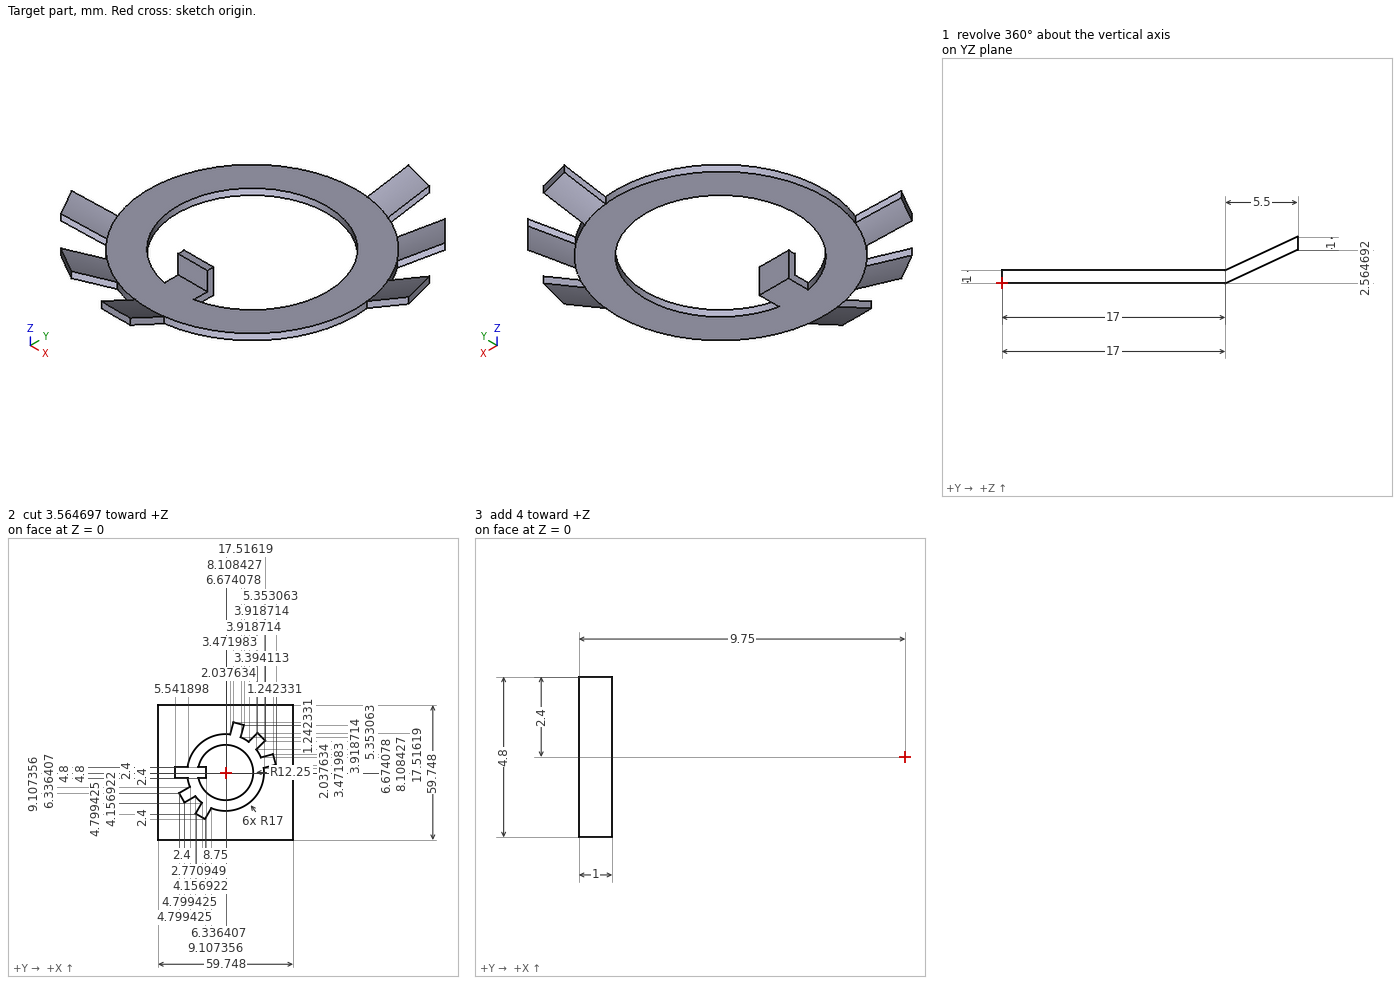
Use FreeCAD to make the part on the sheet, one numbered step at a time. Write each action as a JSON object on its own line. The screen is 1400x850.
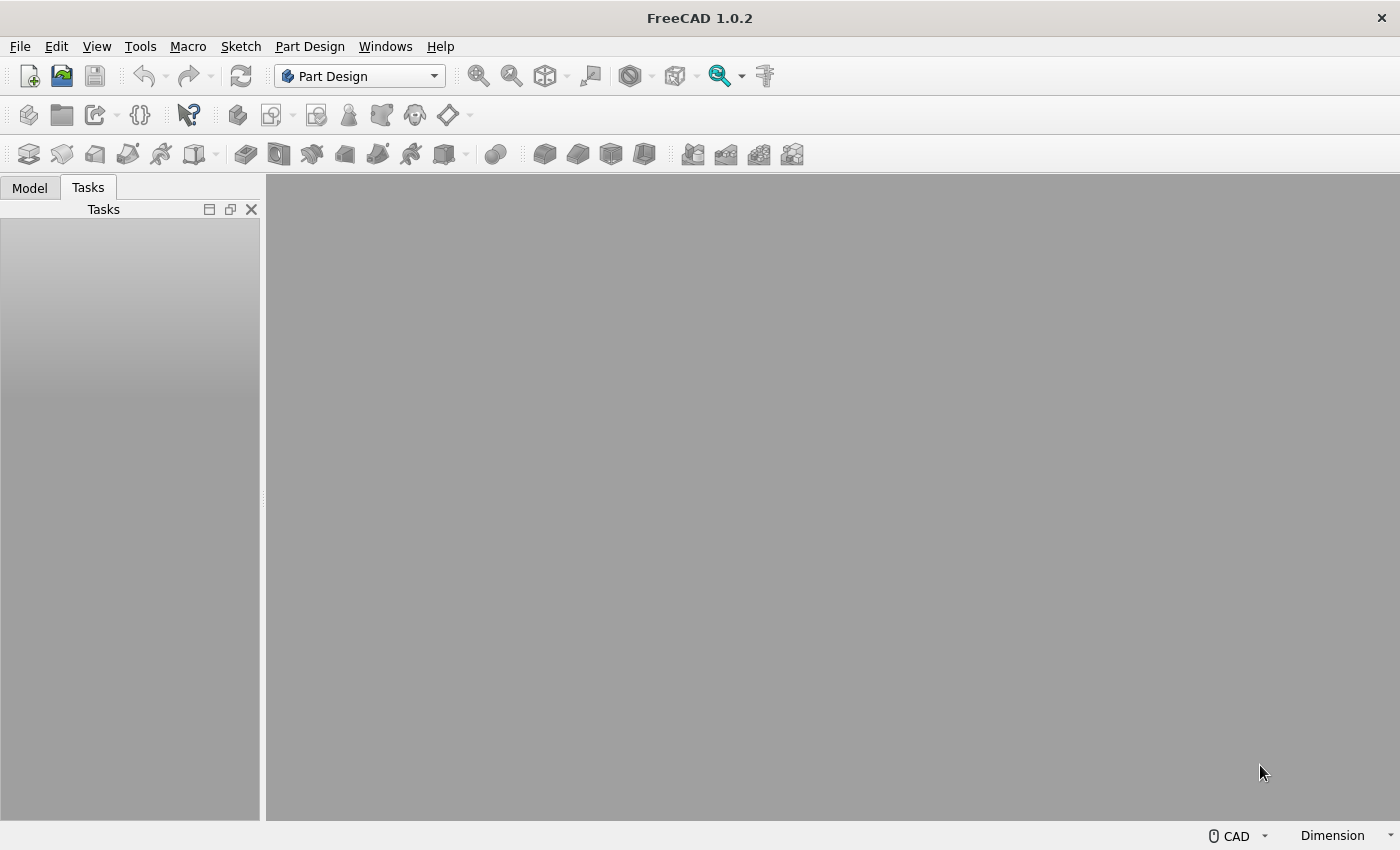
{"action": "left_click", "coordinate": [29, 76]}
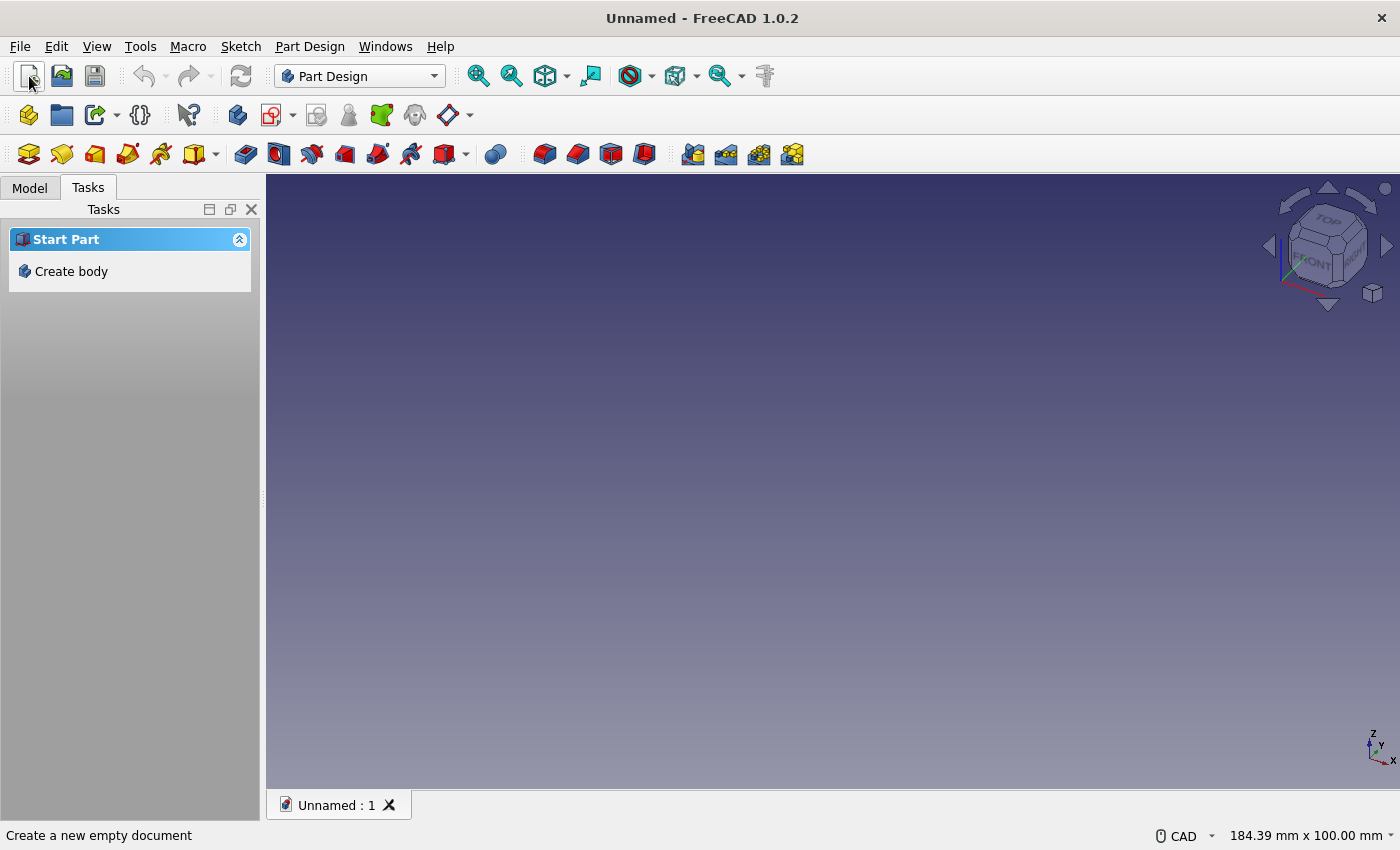
{"action": "left_click", "coordinate": [270, 116]}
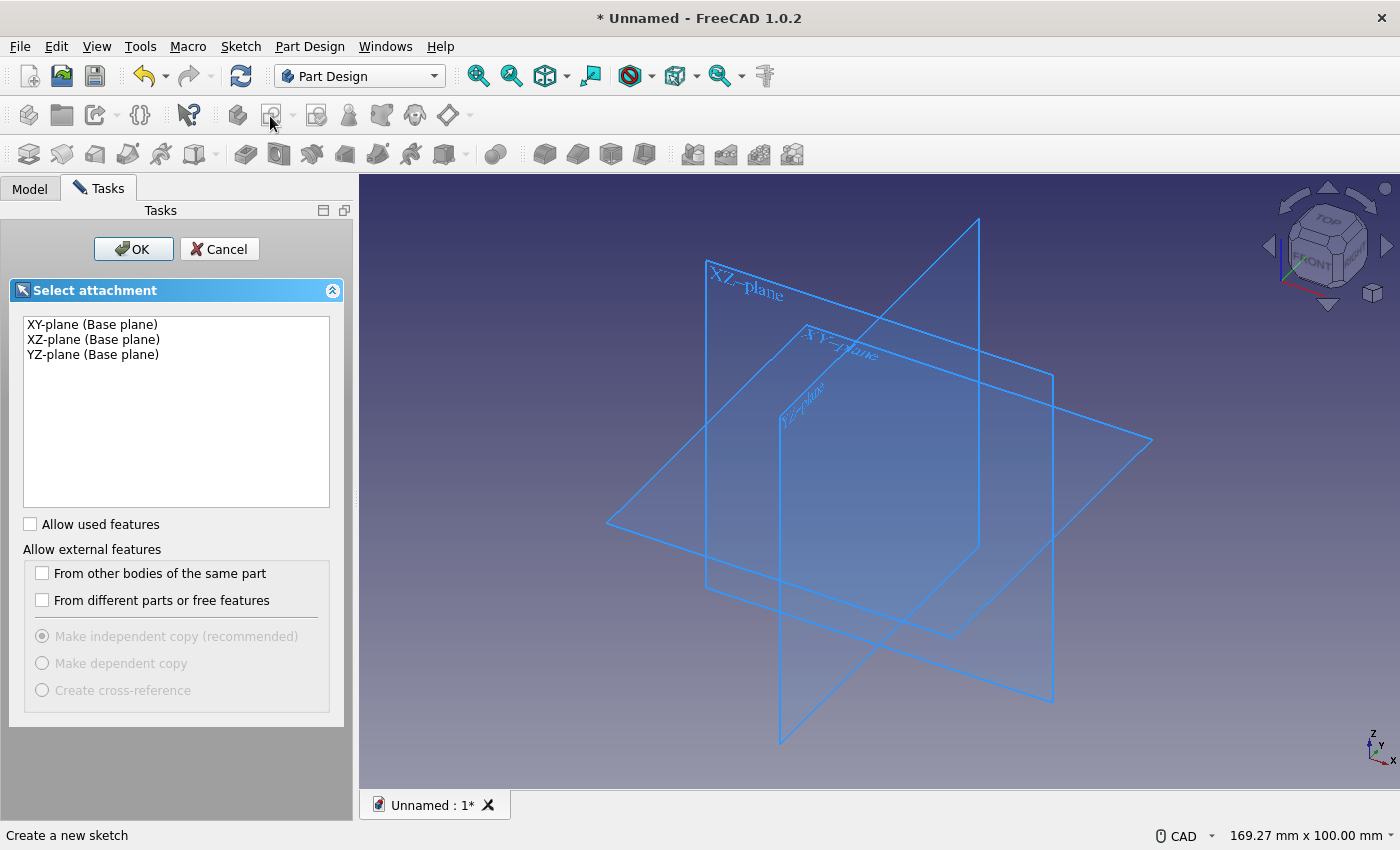
{"action": "left_click", "coordinate": [84, 354]}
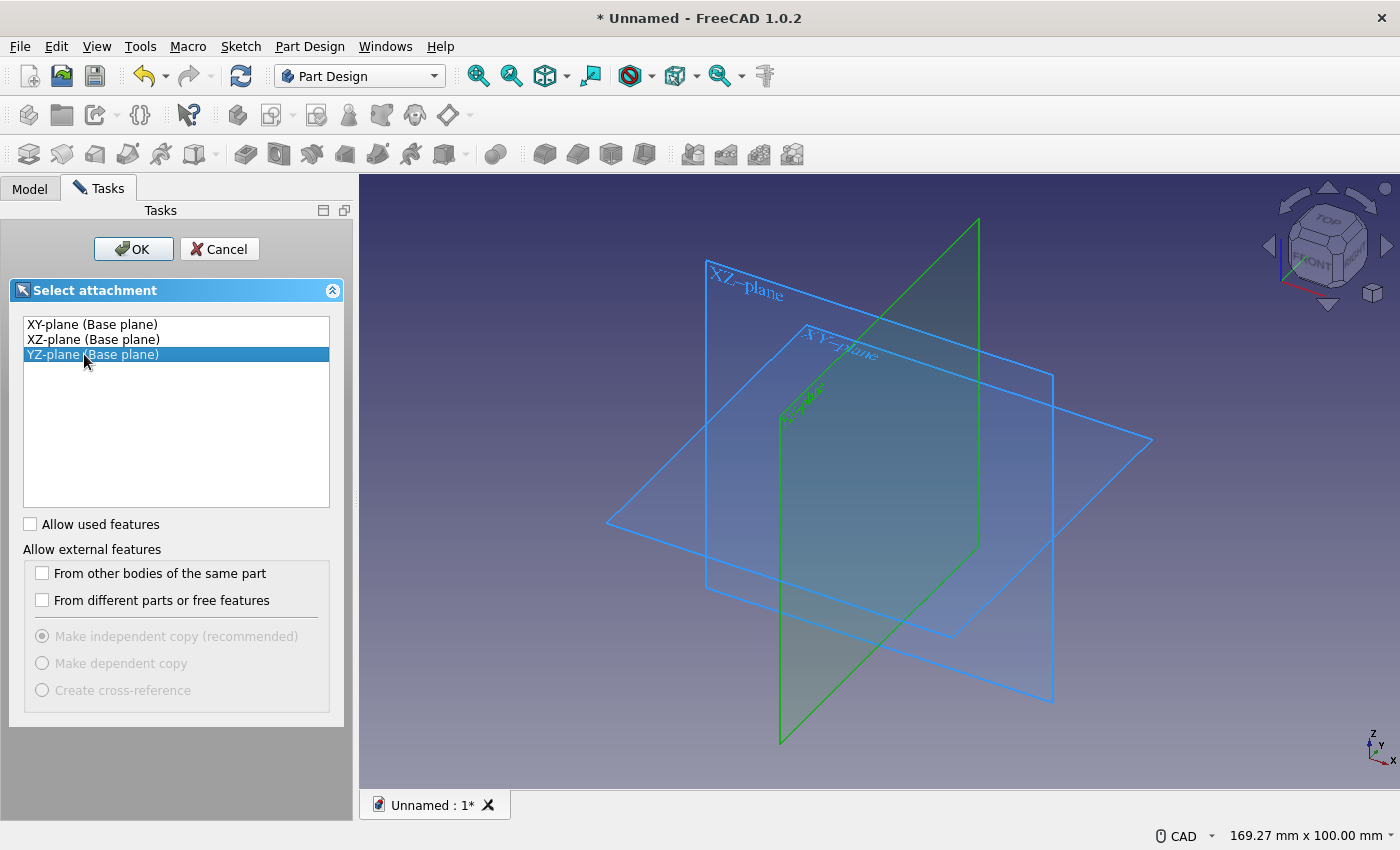
{"action": "left_click", "coordinate": [134, 249]}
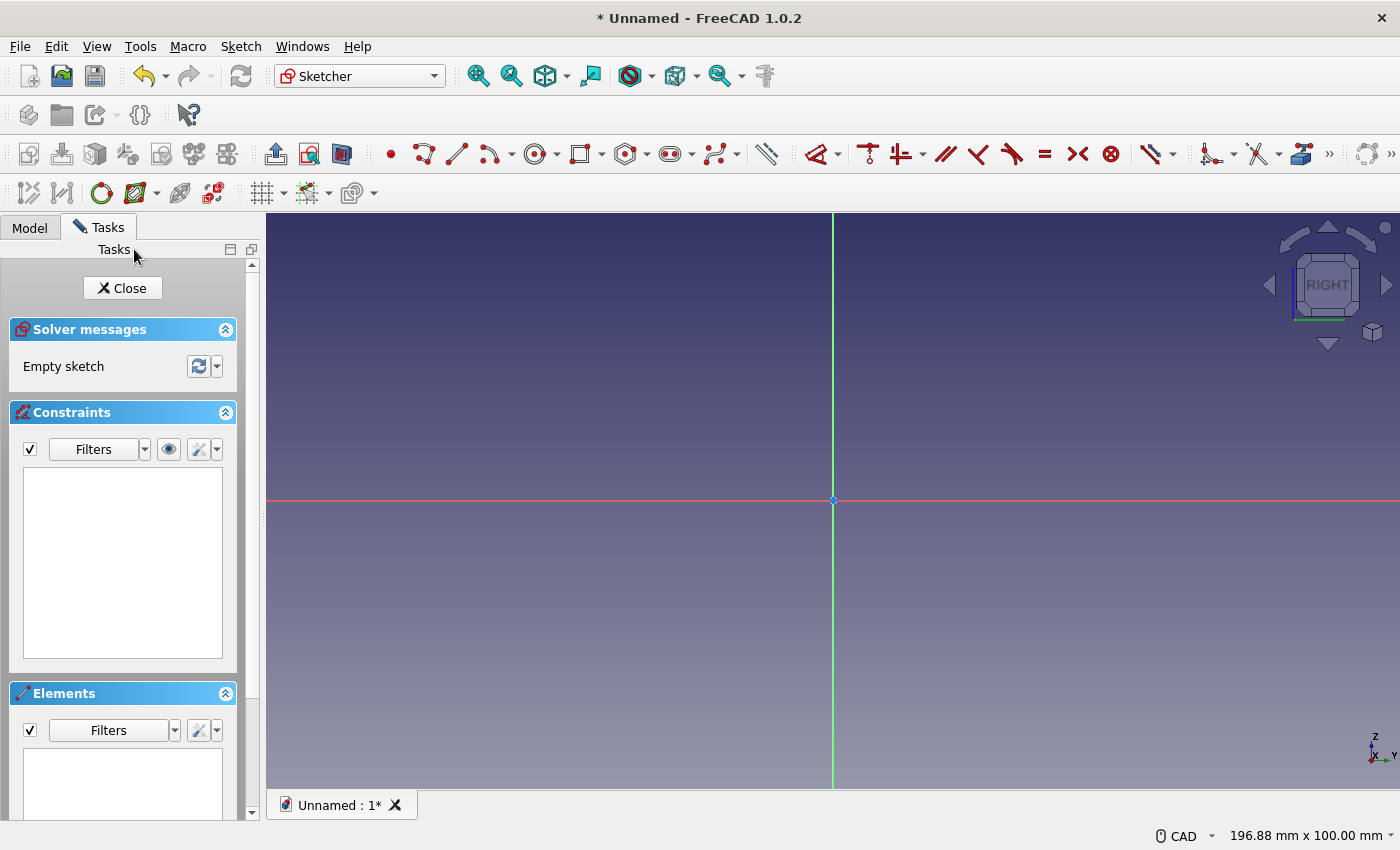
{"action": "scroll", "coordinate": [932, 488], "scroll_direction": "up", "scroll_amount": 8}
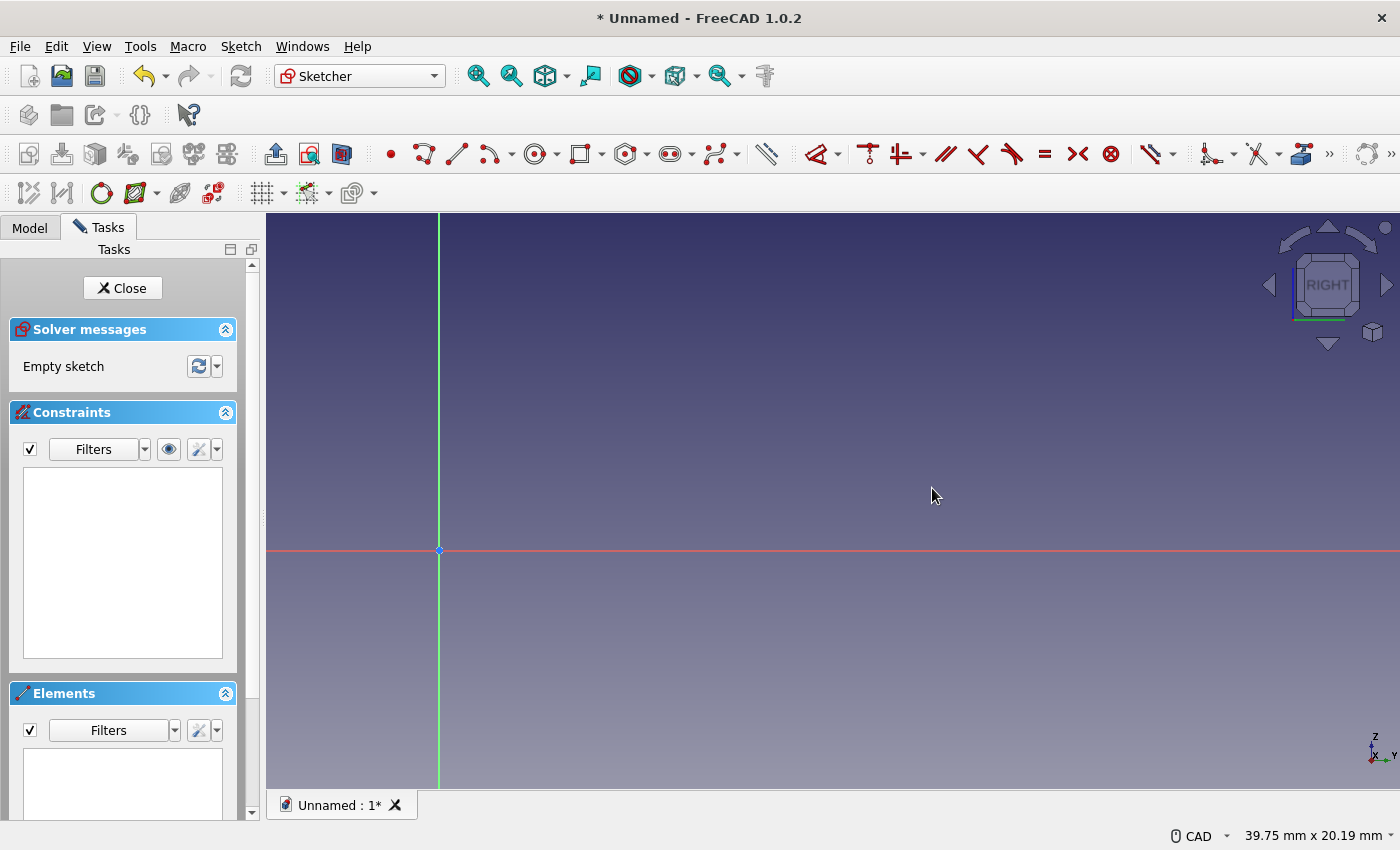
{"action": "left_click", "coordinate": [424, 154]}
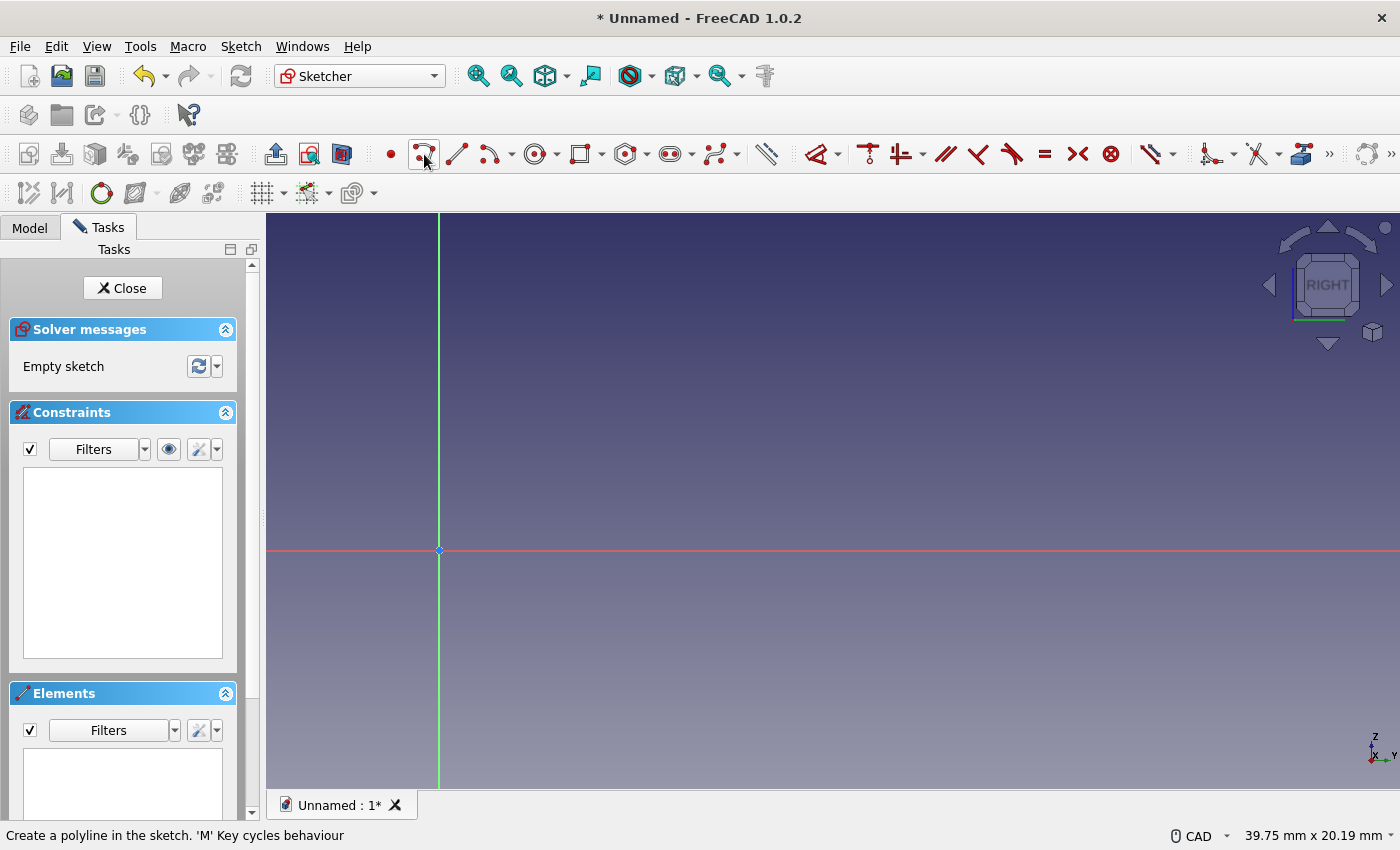
{"action": "left_click", "coordinate": [439, 550]}
{"action": "left_click", "coordinate": [924, 541]}
{"action": "left_click", "coordinate": [1081, 477]}
{"action": "left_click", "coordinate": [1081, 449]}
{"action": "left_click", "coordinate": [924, 522]}
{"action": "left_click", "coordinate": [448, 522]}
{"action": "left_click", "coordinate": [439, 550]}
{"action": "key", "text": "Escape"}
{"action": "key", "text": "Escape"}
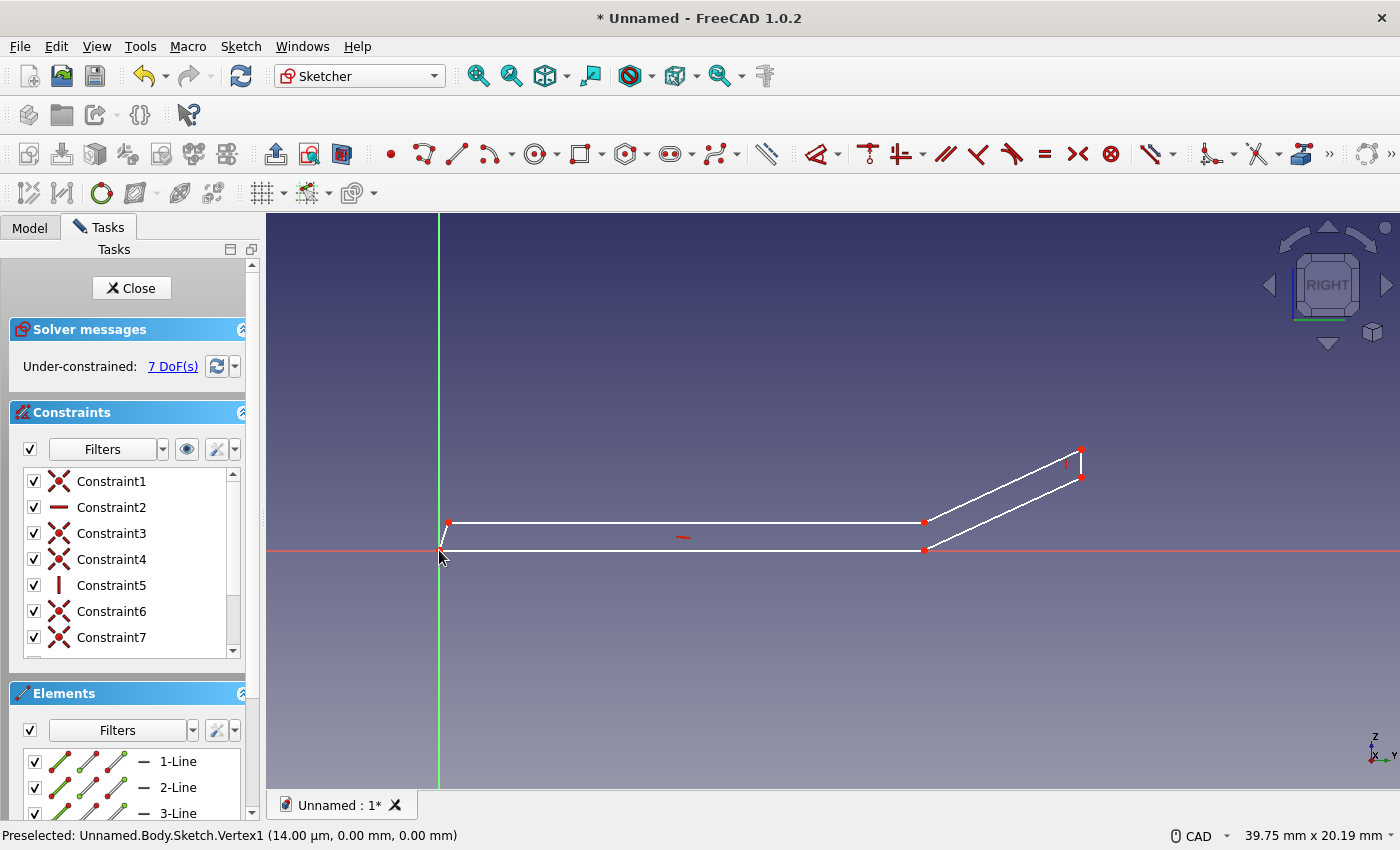
{"action": "scroll", "coordinate": [443, 539], "scroll_direction": "up", "scroll_amount": 2}